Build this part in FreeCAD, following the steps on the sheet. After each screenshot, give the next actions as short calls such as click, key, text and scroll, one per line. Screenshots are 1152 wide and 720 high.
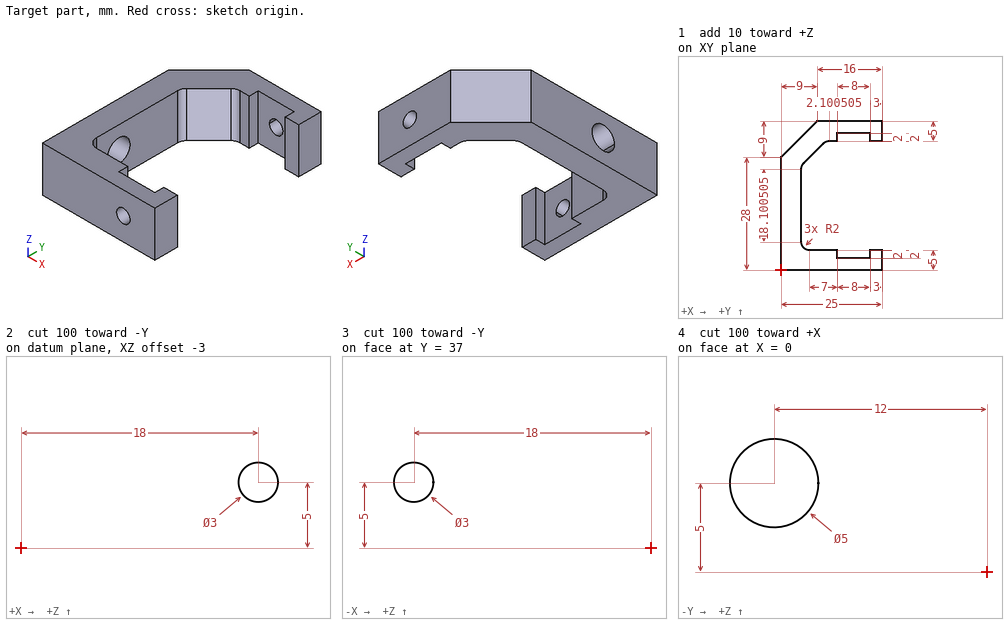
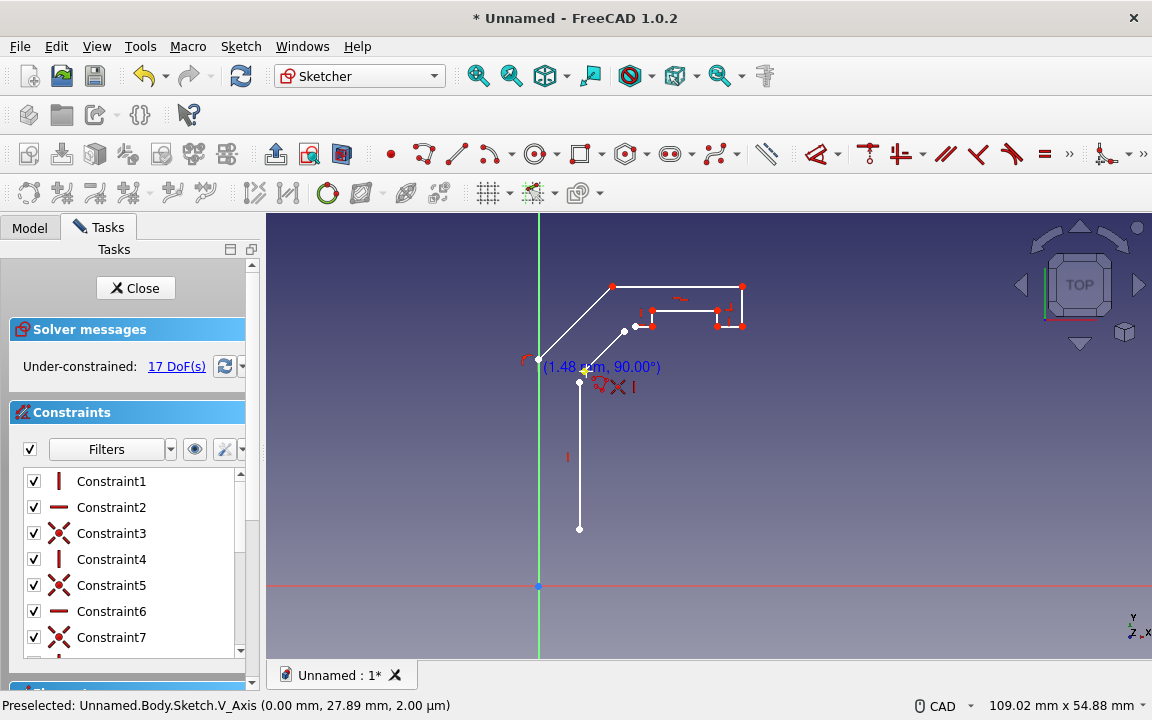
click(539, 586)
click(742, 577)
click(742, 546)
click(718, 546)
click(718, 562)
click(653, 562)
click(653, 546)
click(596, 546)
right_click(596, 546)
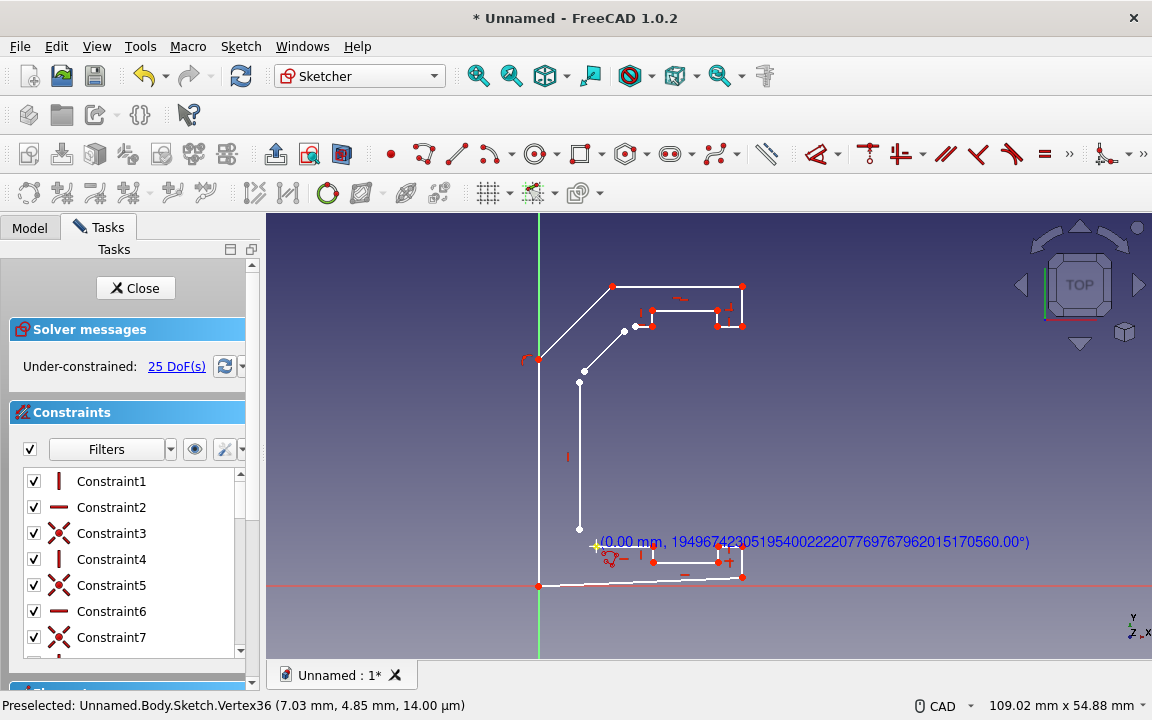
key(g)
key(3)
key(a)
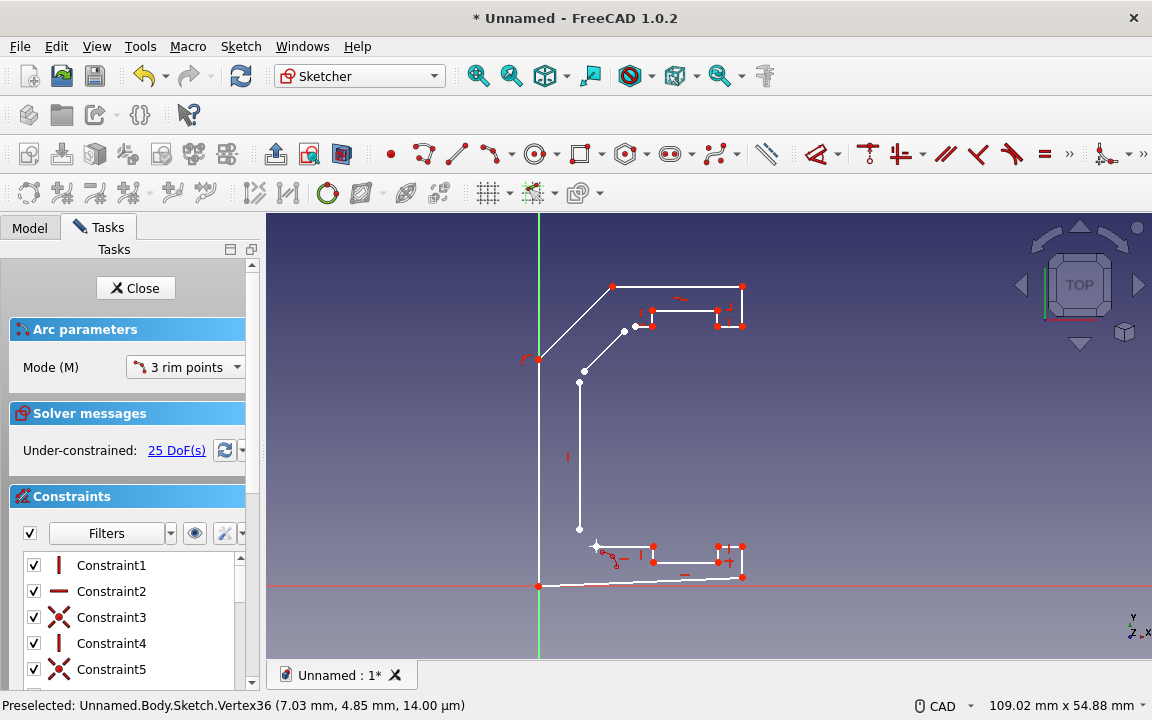
scroll(580, 382, up, 2)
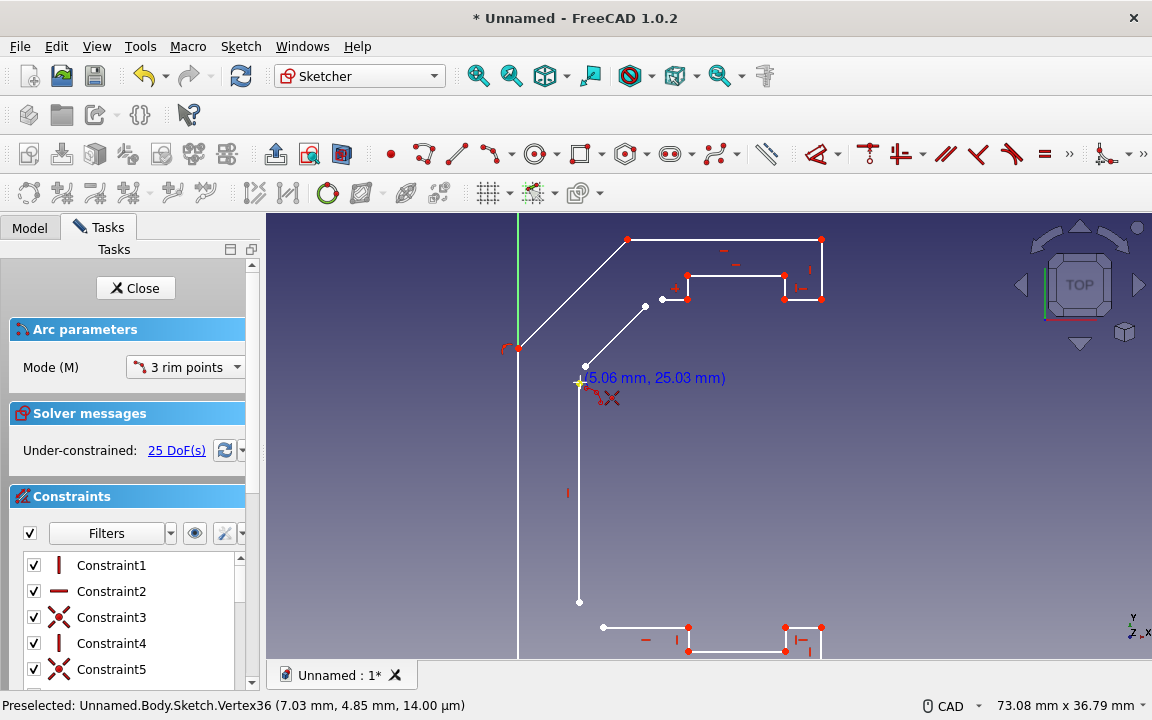
click(579, 383)
click(586, 367)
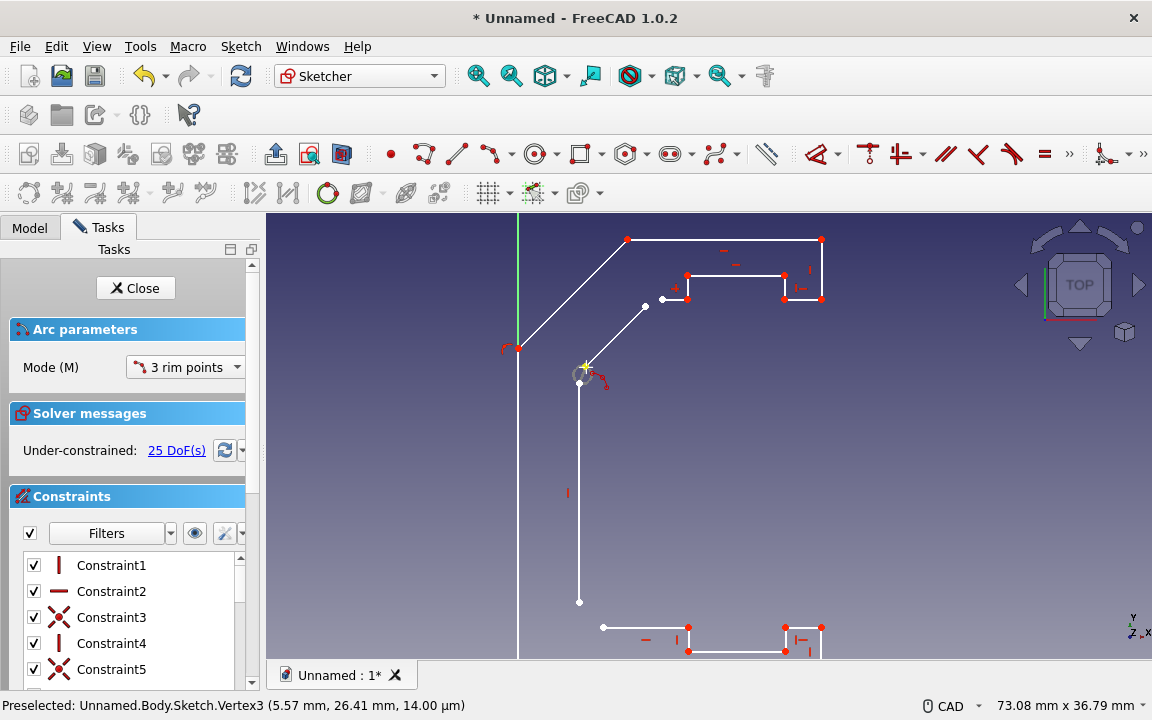
scroll(581, 373, up, 11)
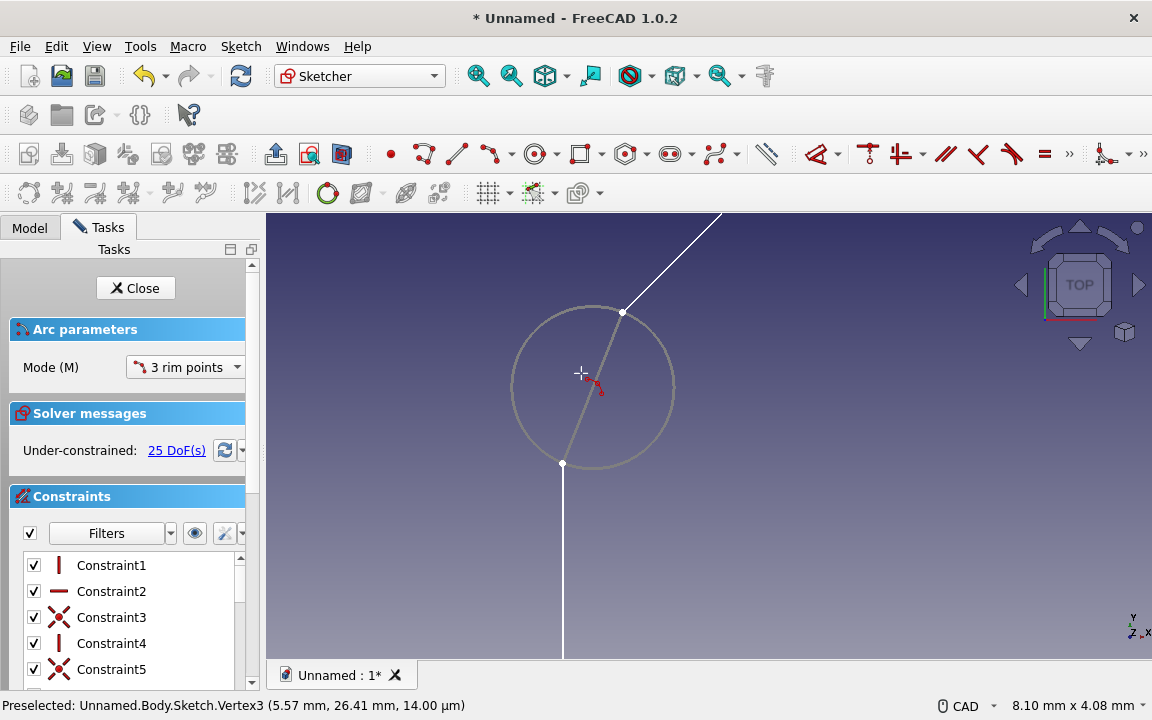
click(578, 371)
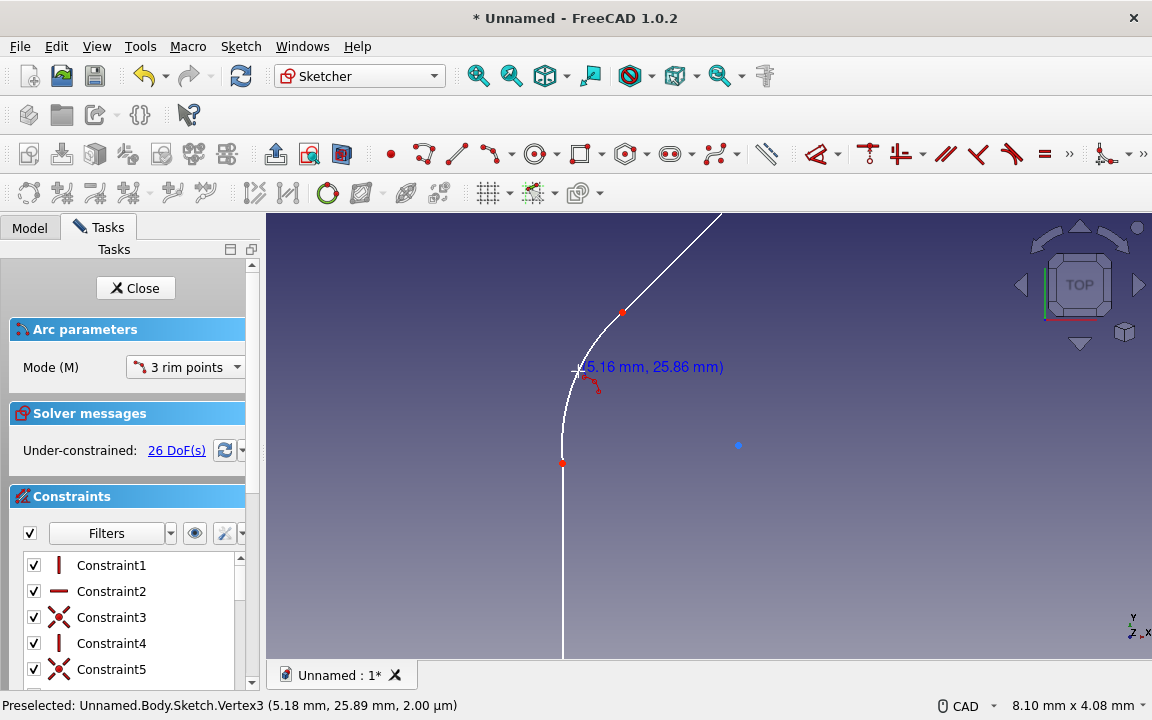
scroll(581, 377, down, 13)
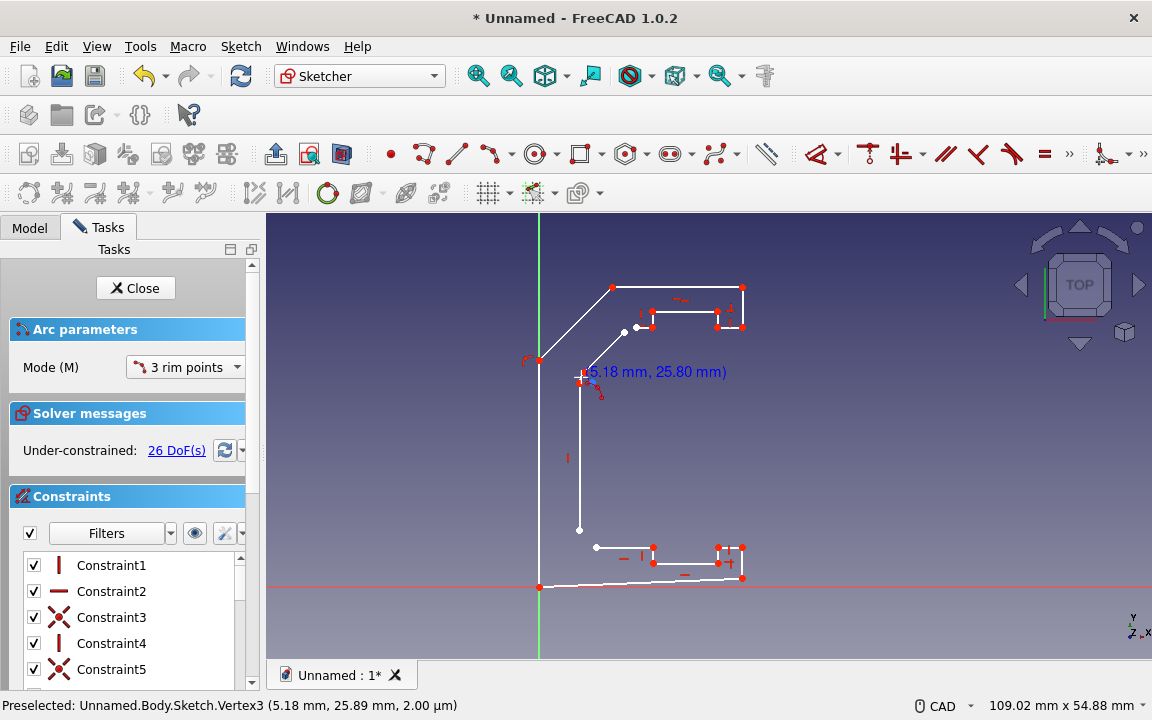
scroll(624, 332, up, 2)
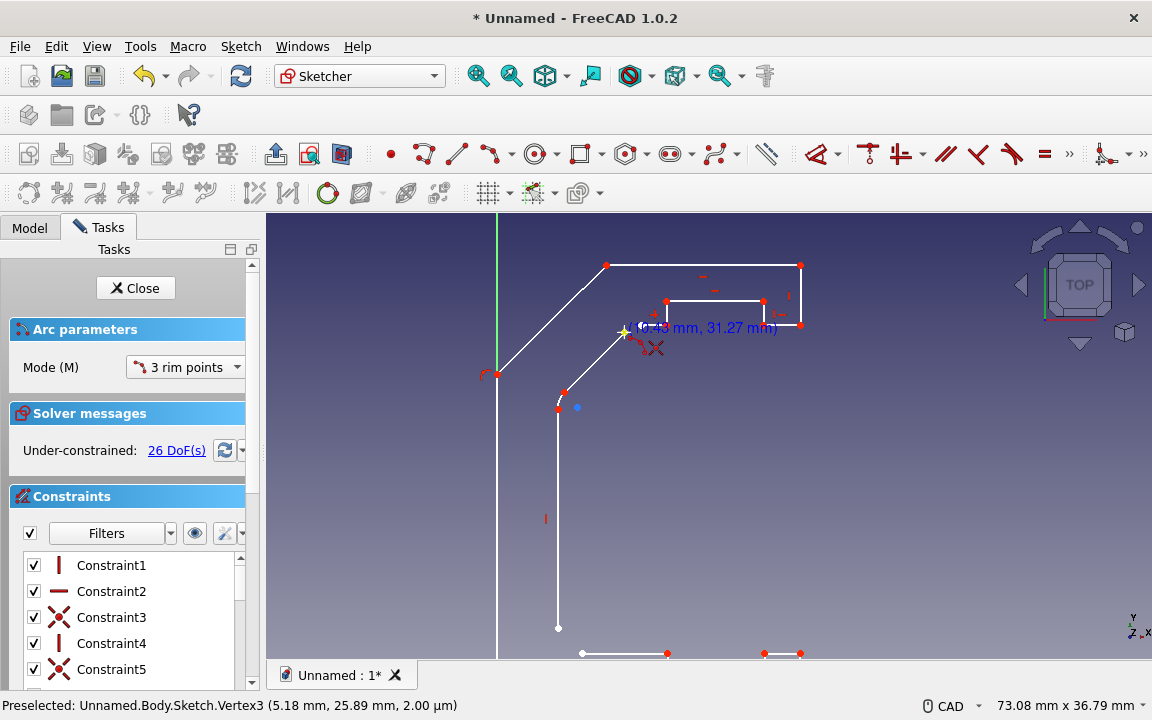
click(625, 332)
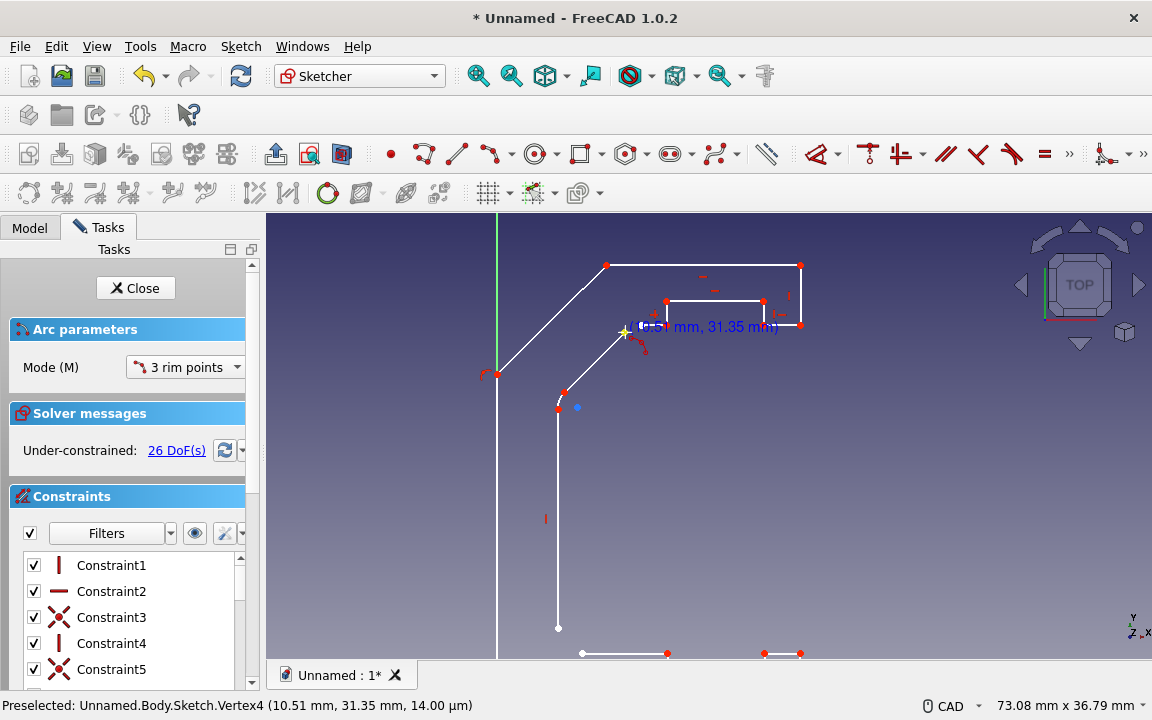
scroll(642, 324, up, 2)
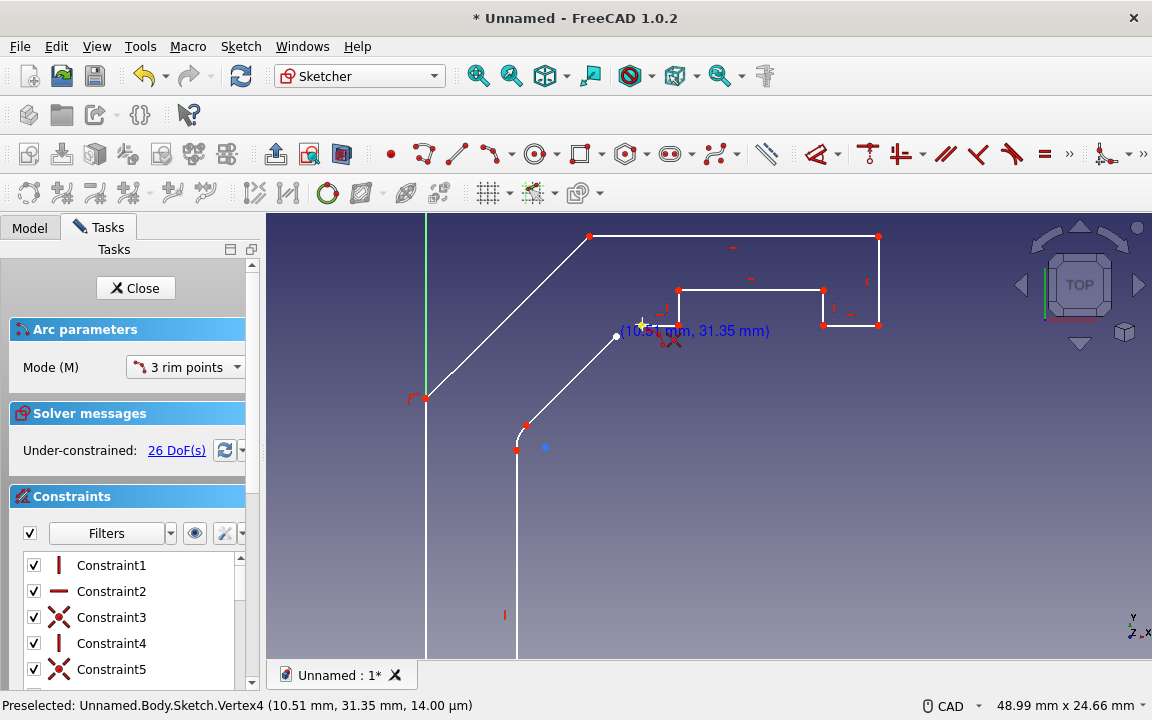
click(641, 326)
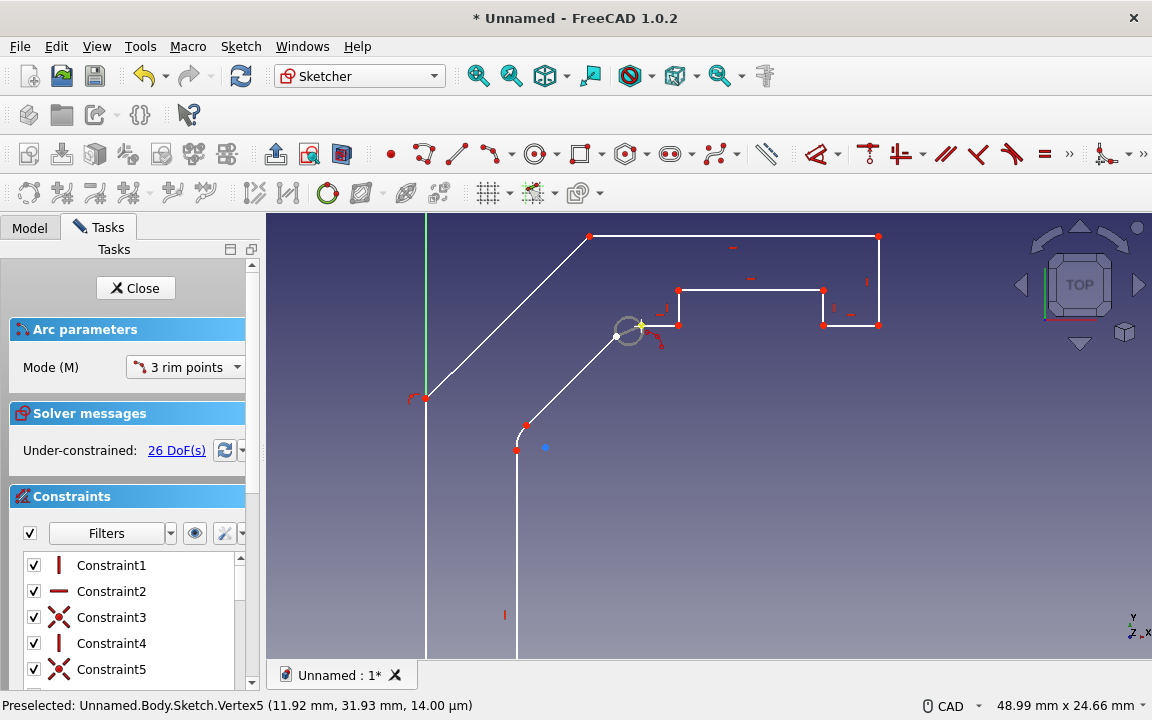
scroll(627, 327, up, 9)